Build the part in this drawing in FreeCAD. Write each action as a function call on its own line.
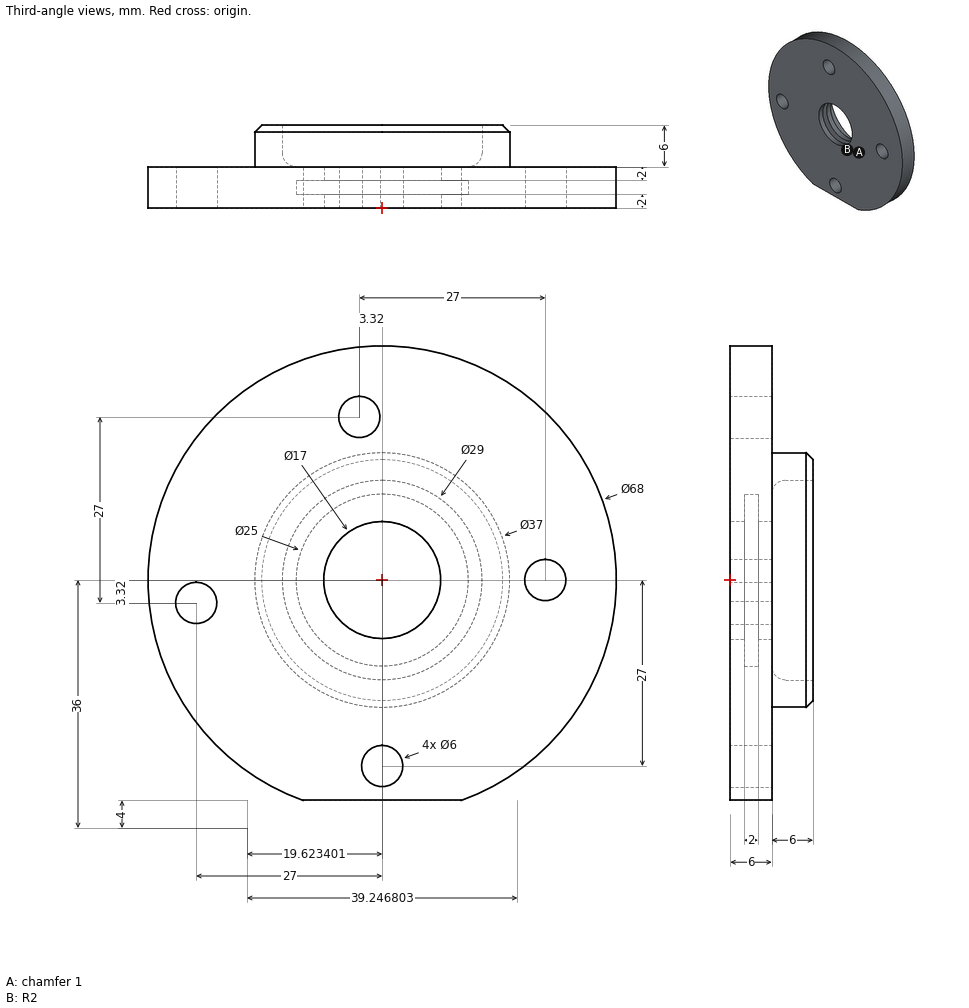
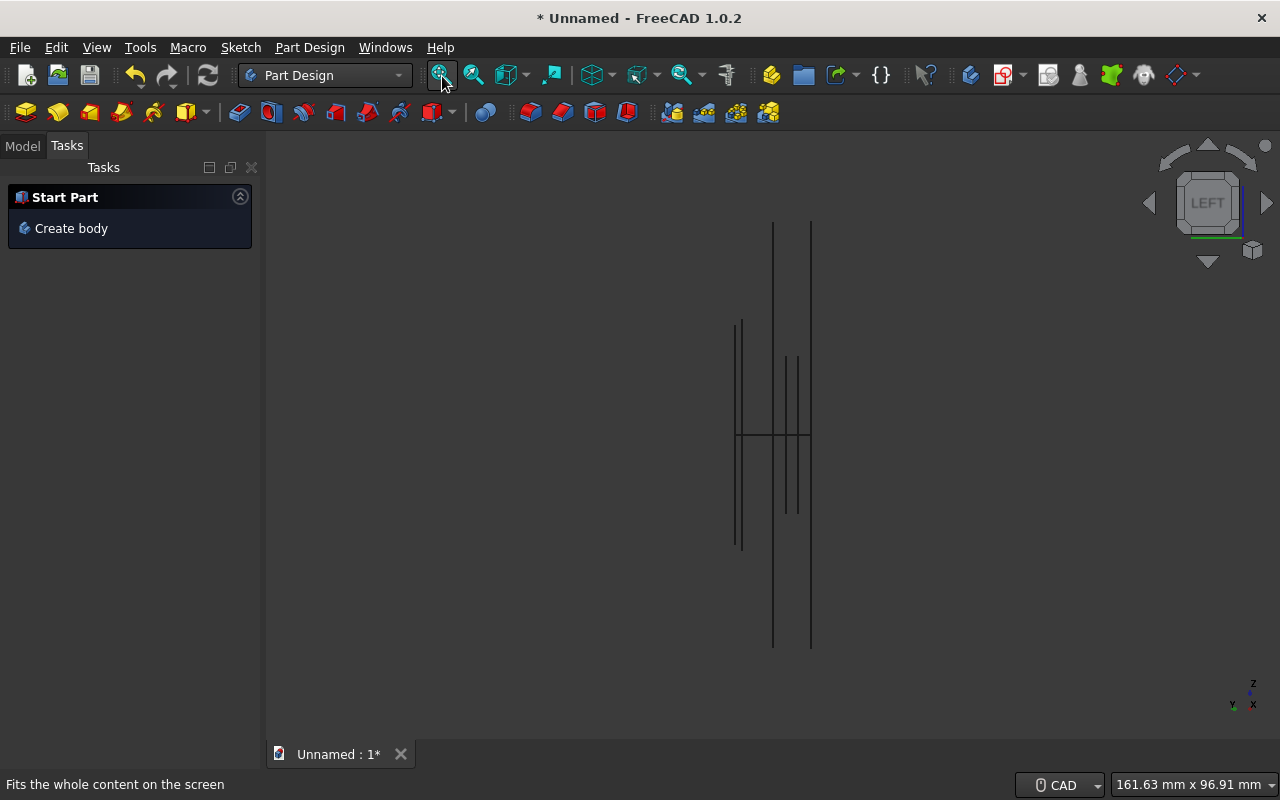
key(0)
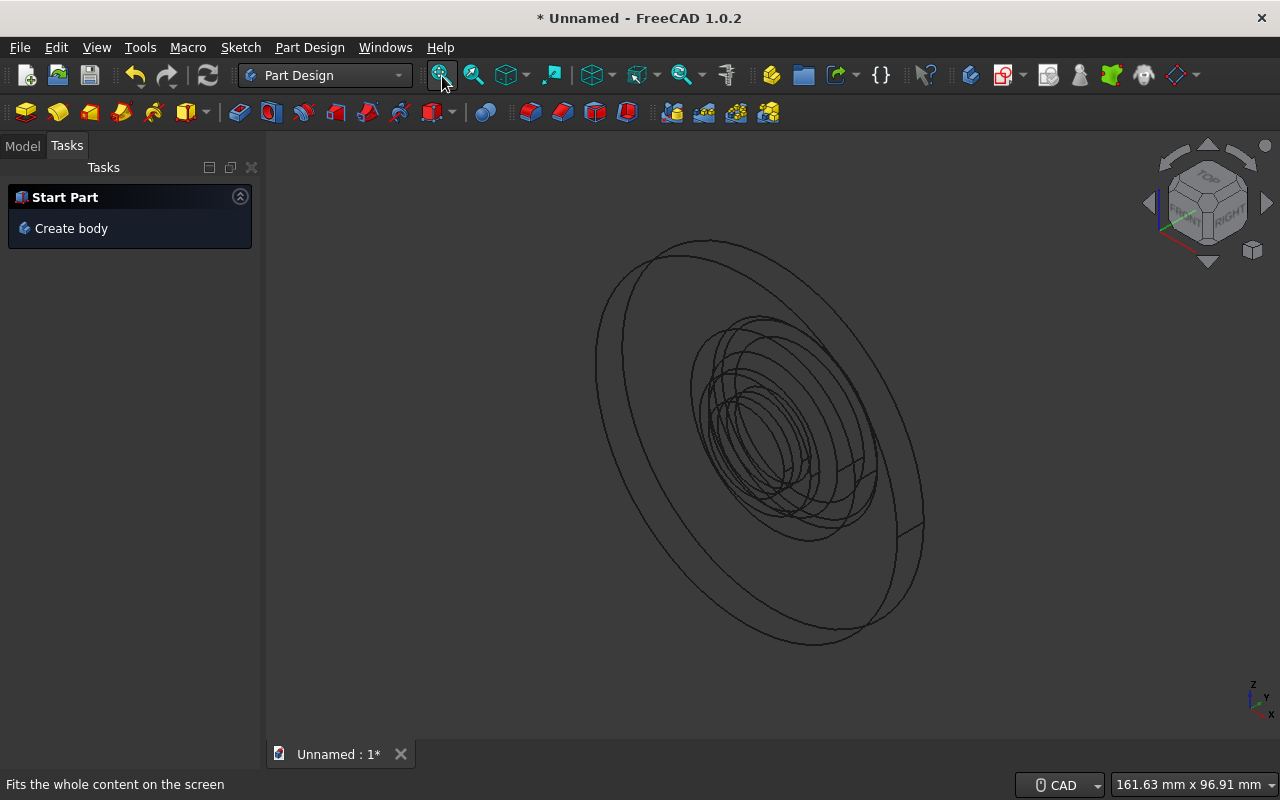
click(721, 360)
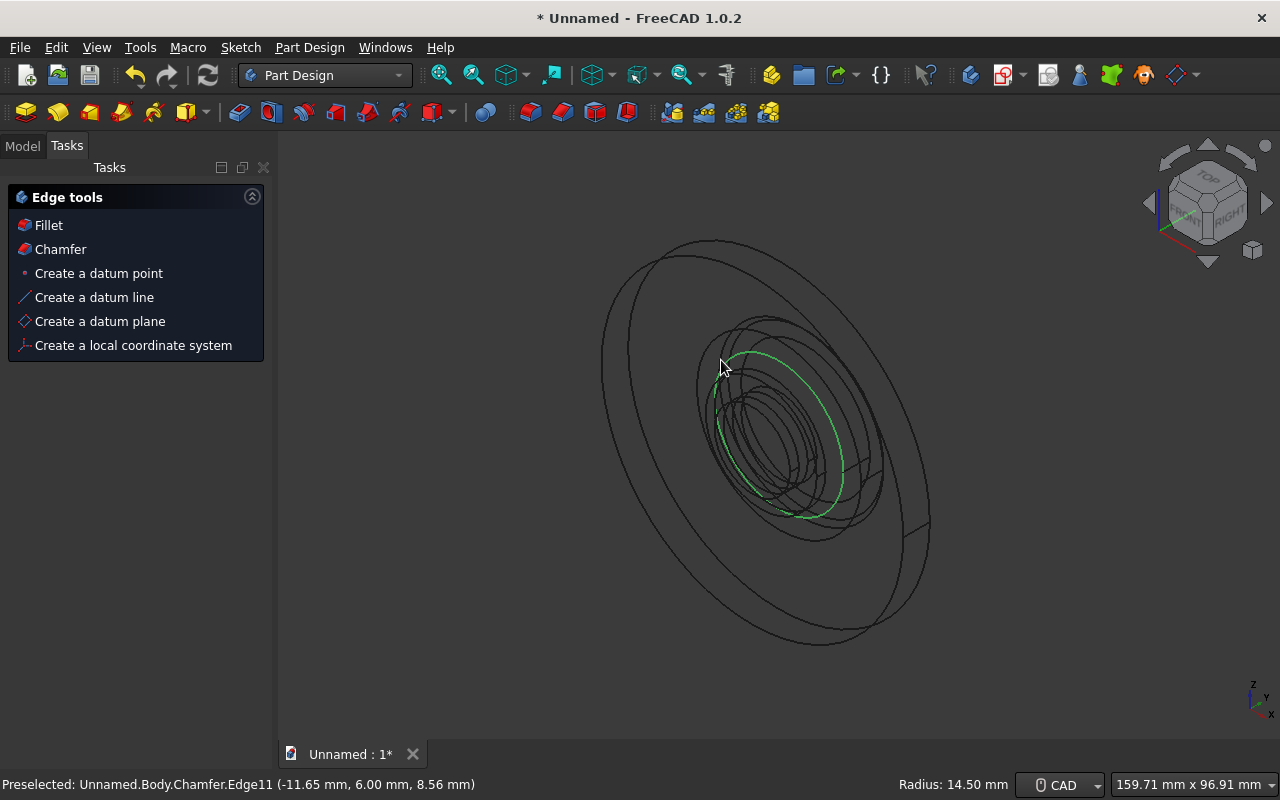
key(v)
key(1)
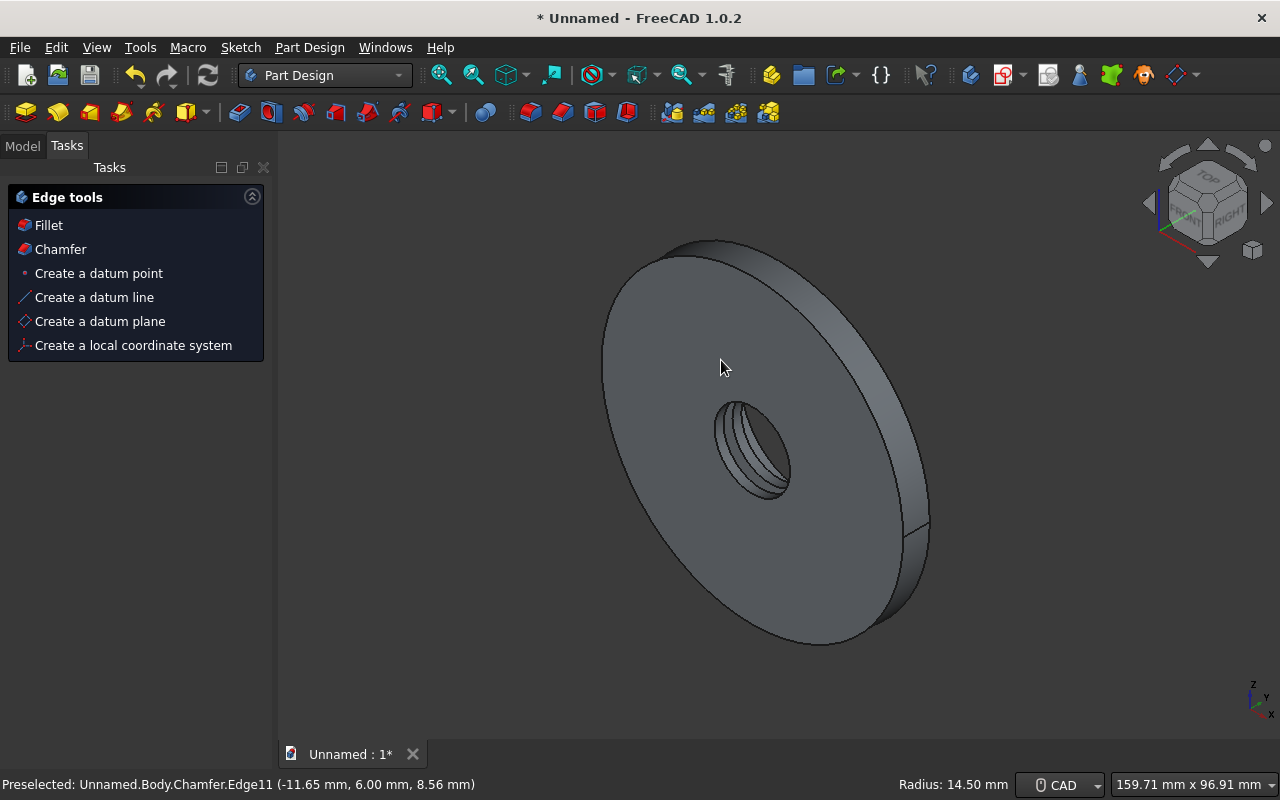
click(532, 112)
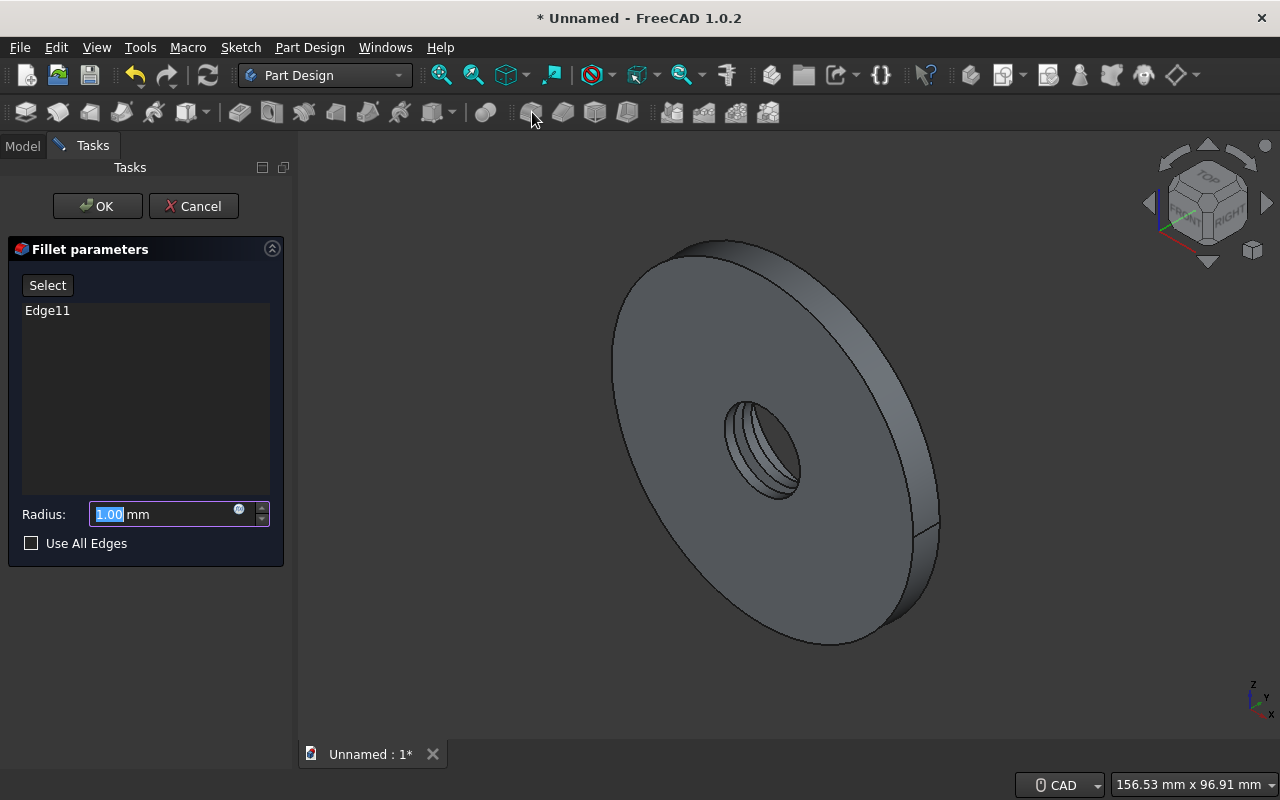
text(2)
key(Tab)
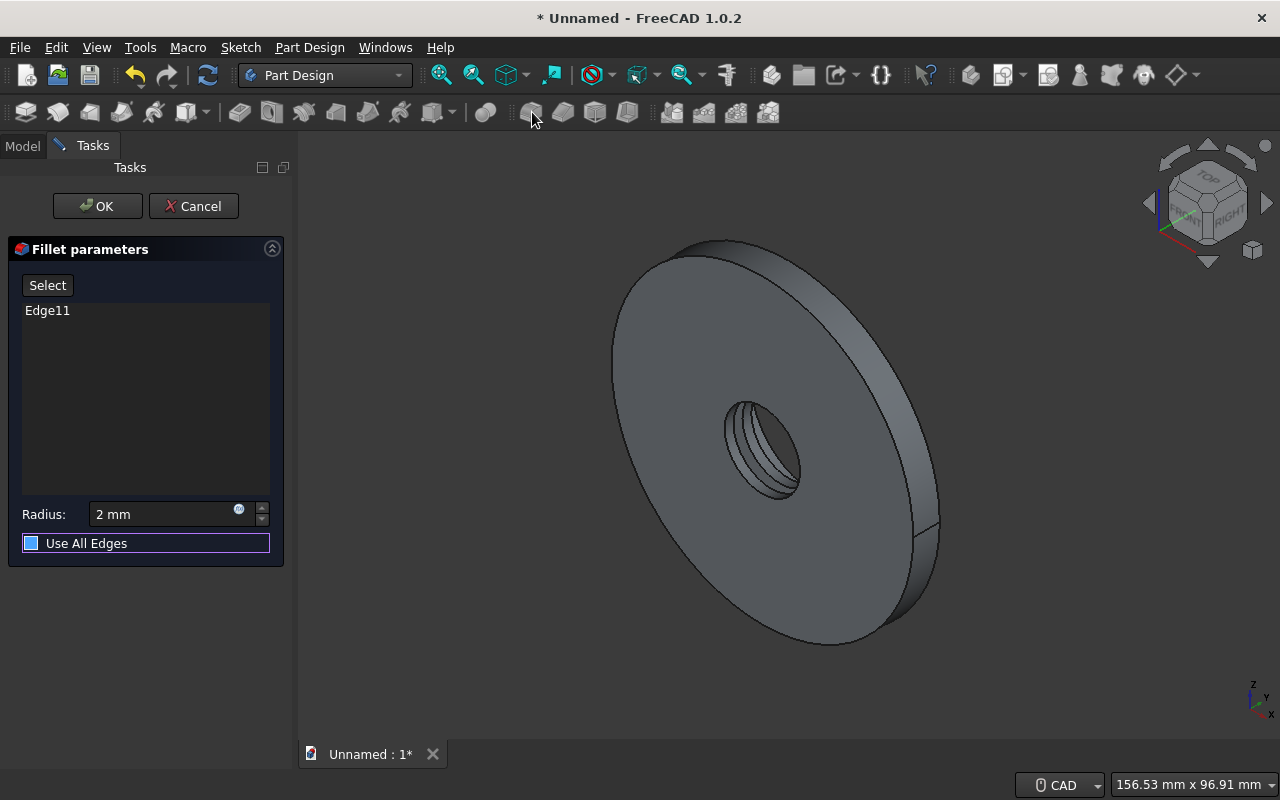
click(98, 206)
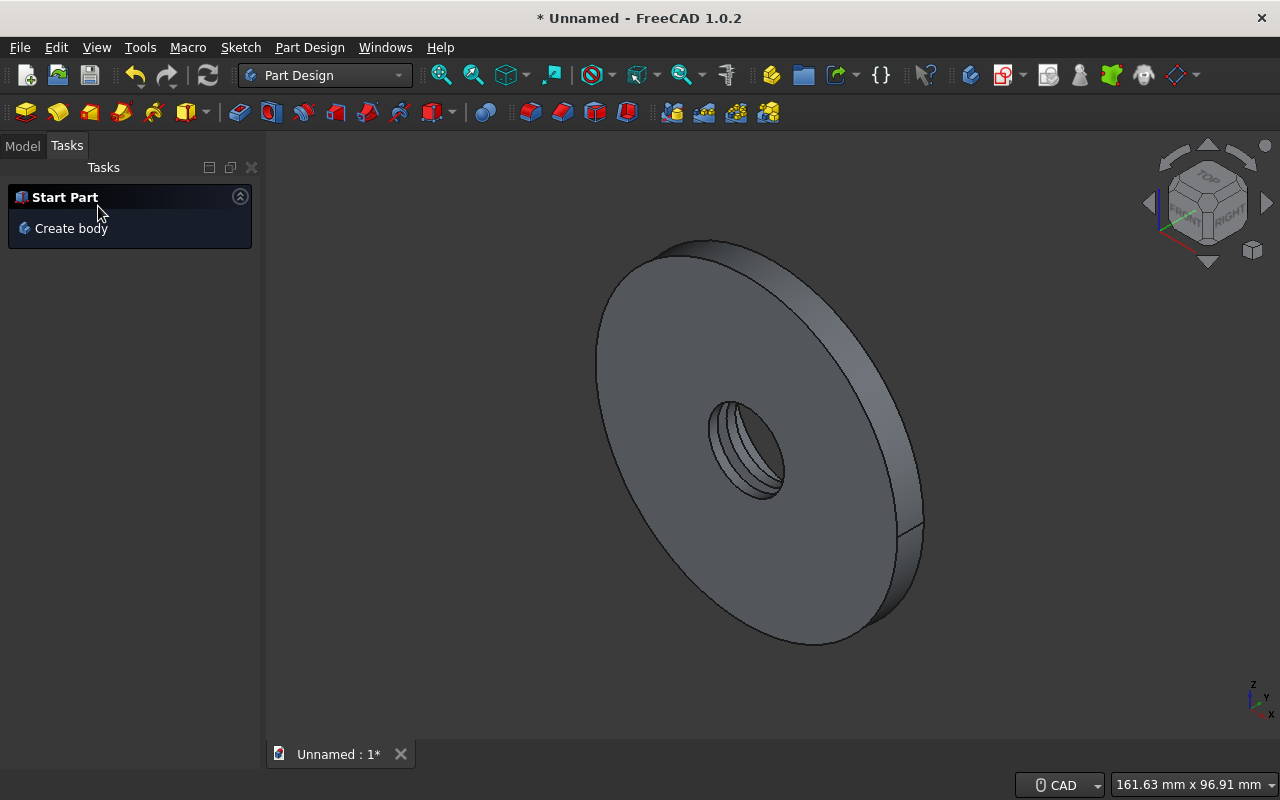
key(4)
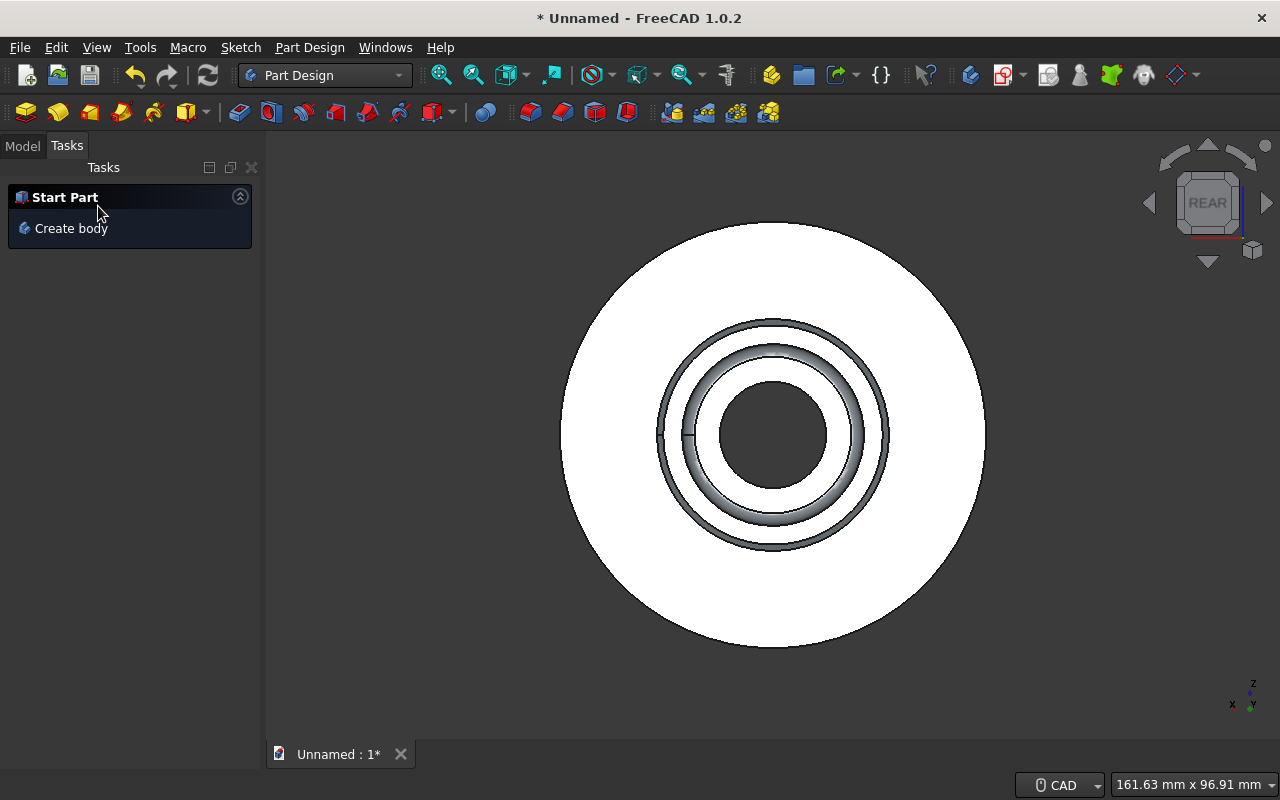
click(651, 556)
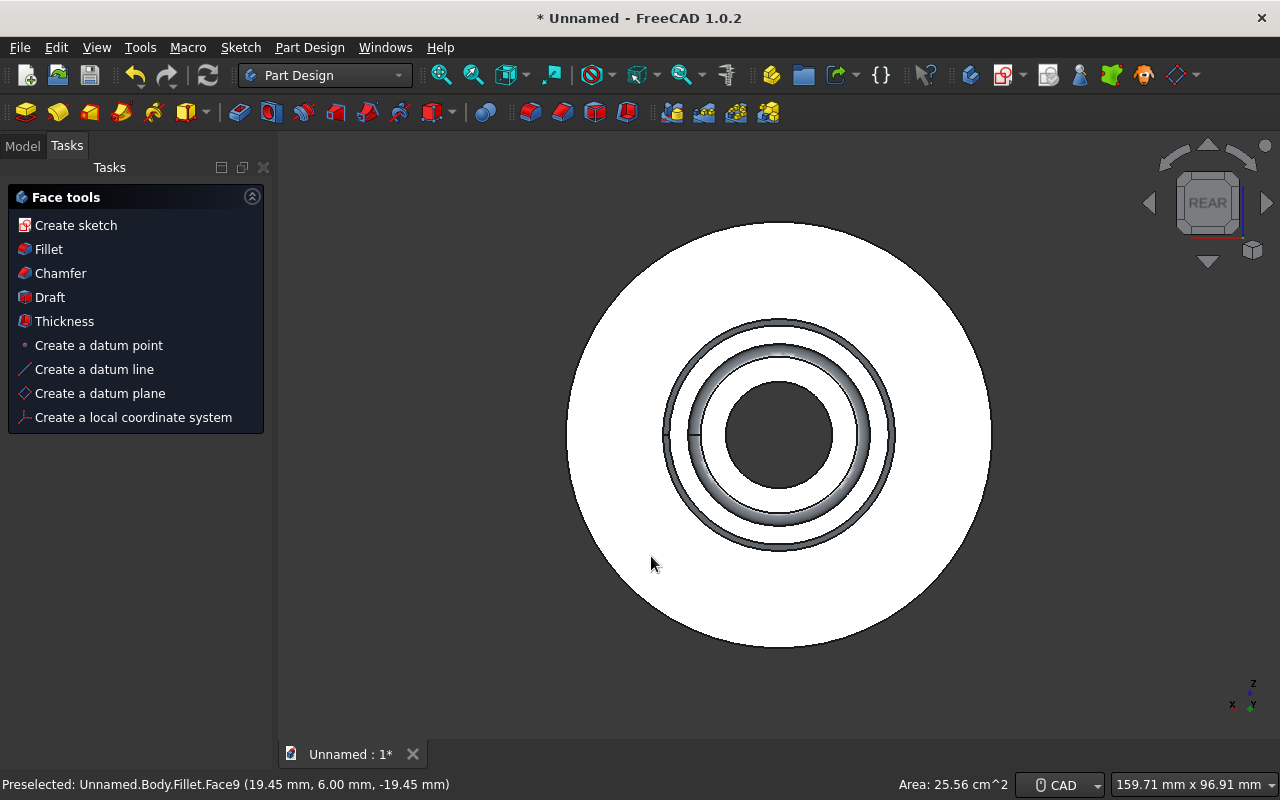
click(1004, 76)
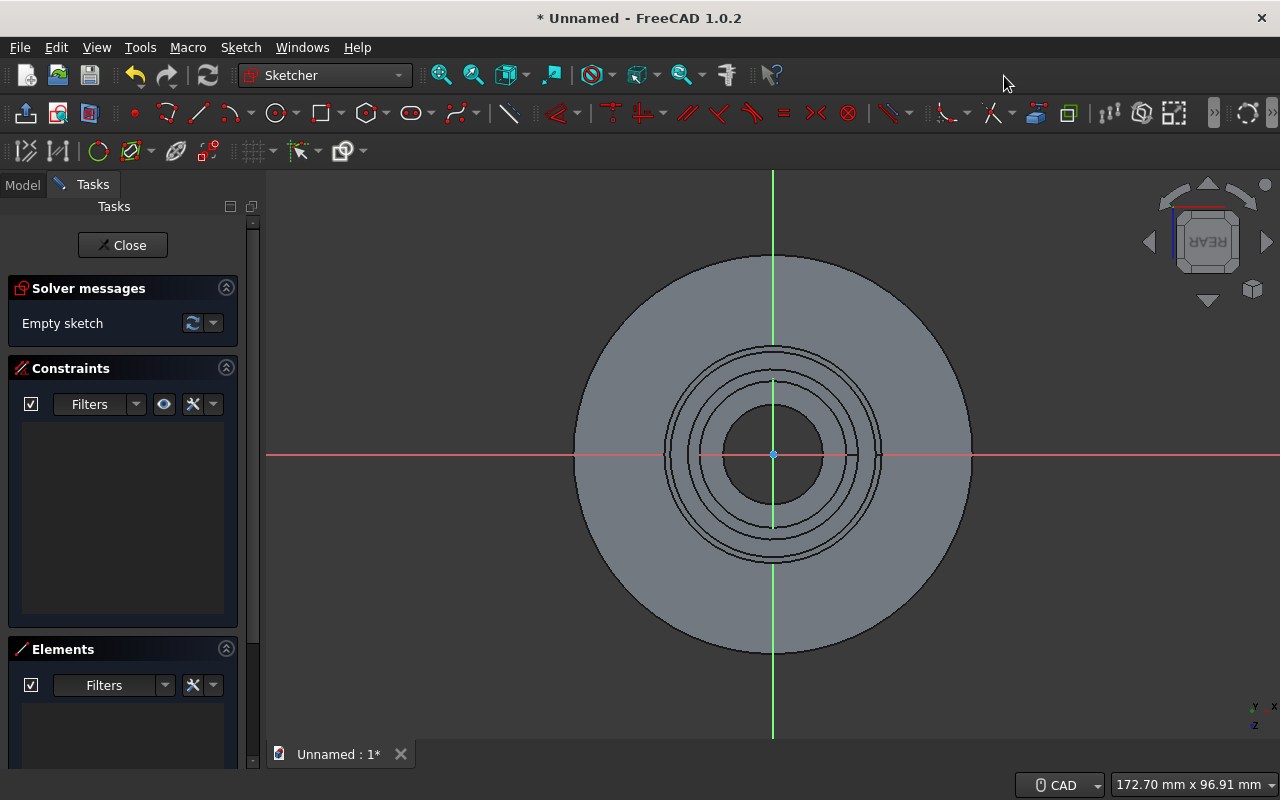
scroll(856, 220, up, 3)